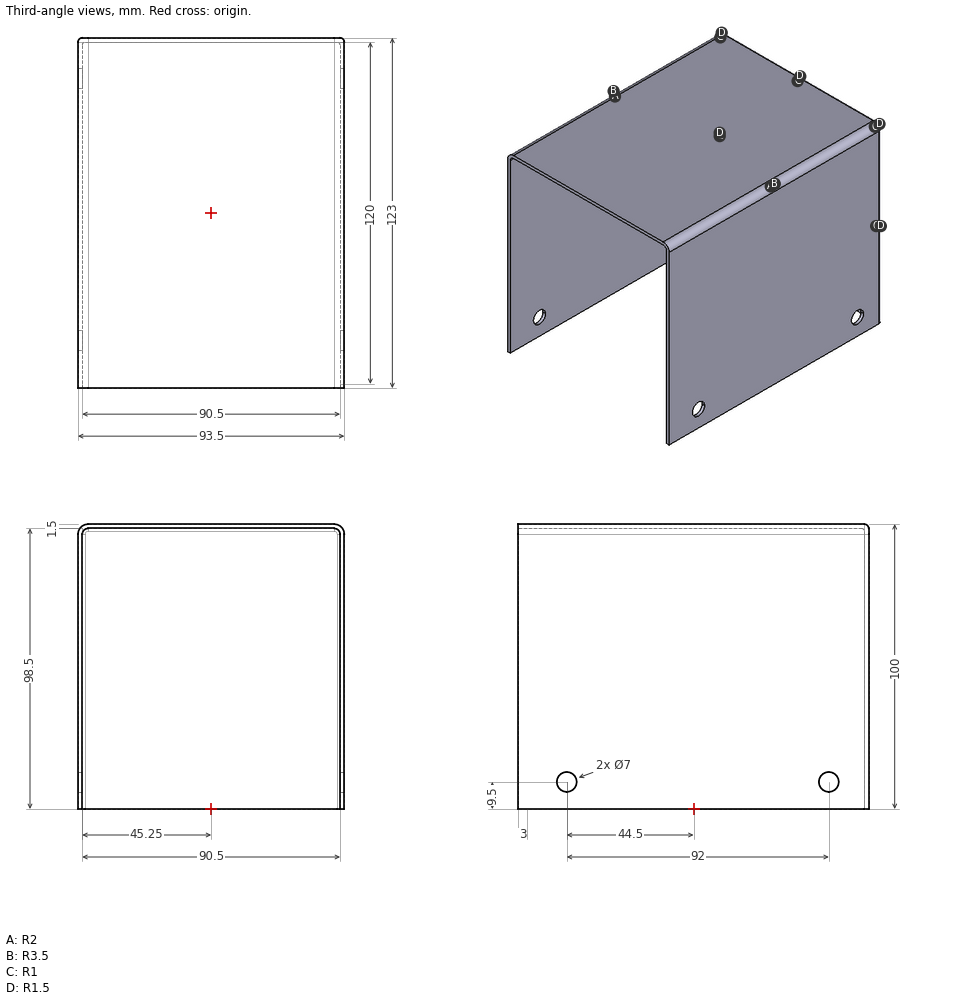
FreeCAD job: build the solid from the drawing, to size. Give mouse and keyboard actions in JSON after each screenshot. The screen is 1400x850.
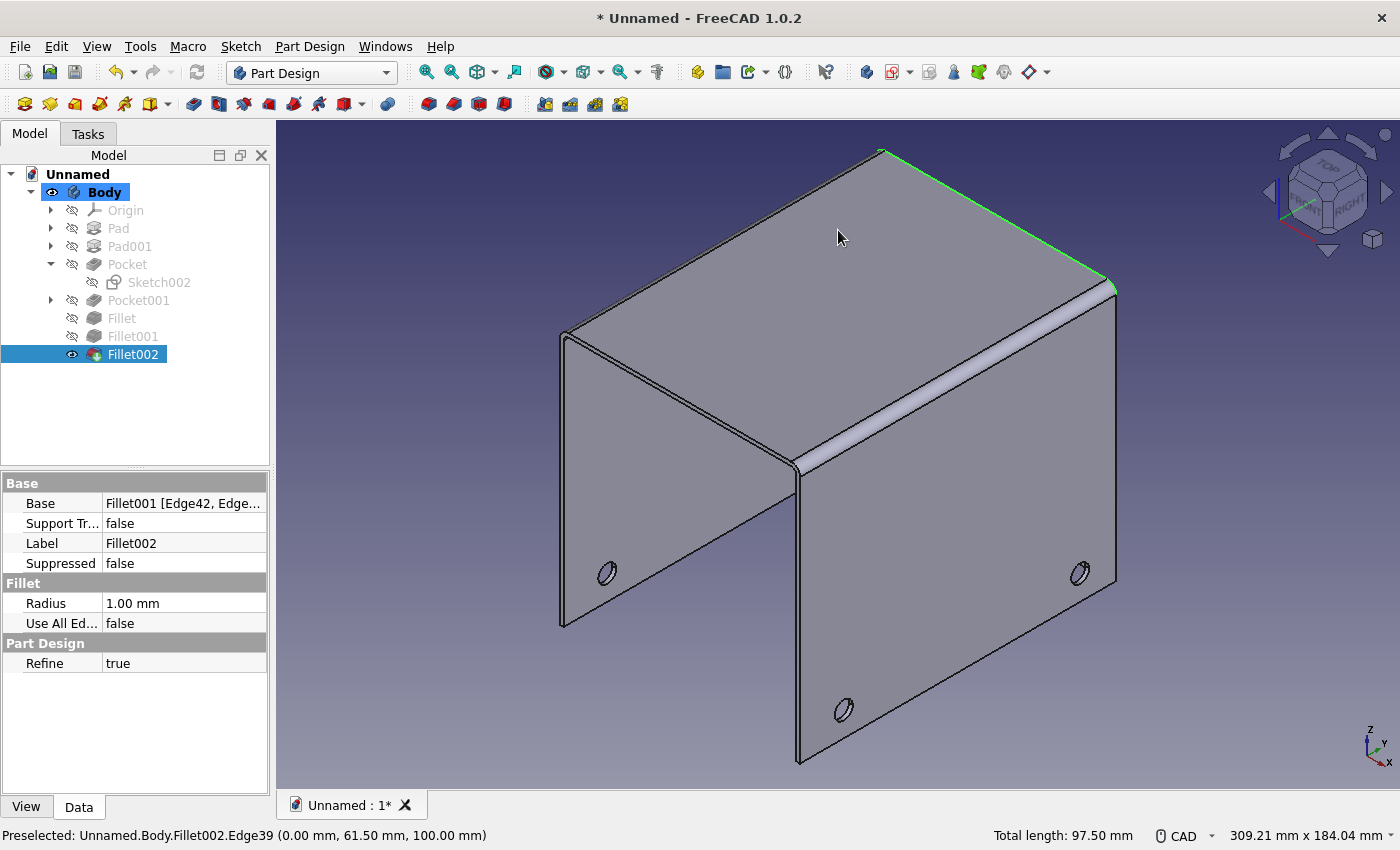
{"action": "key", "text": "1"}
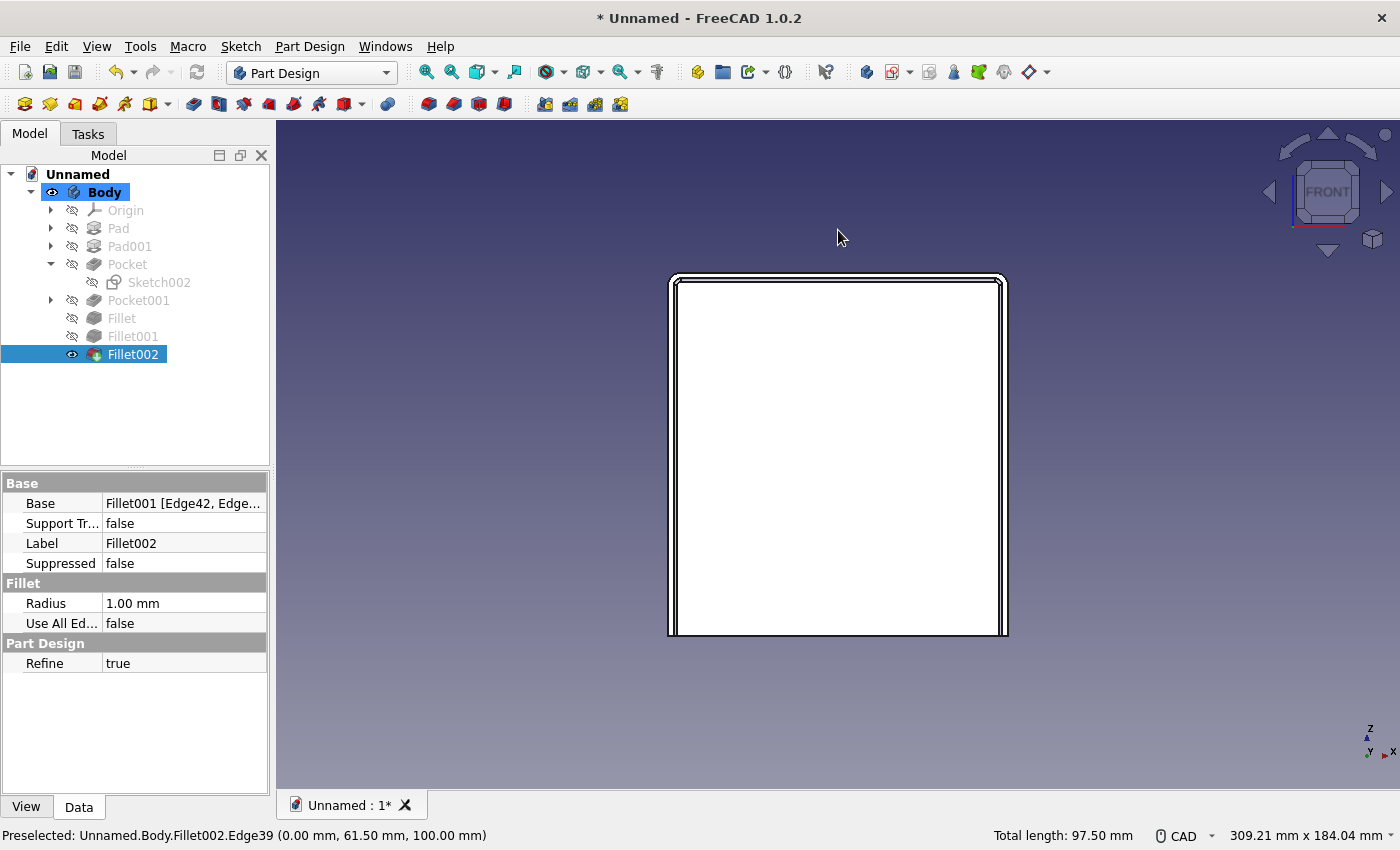
{"action": "key", "text": "3"}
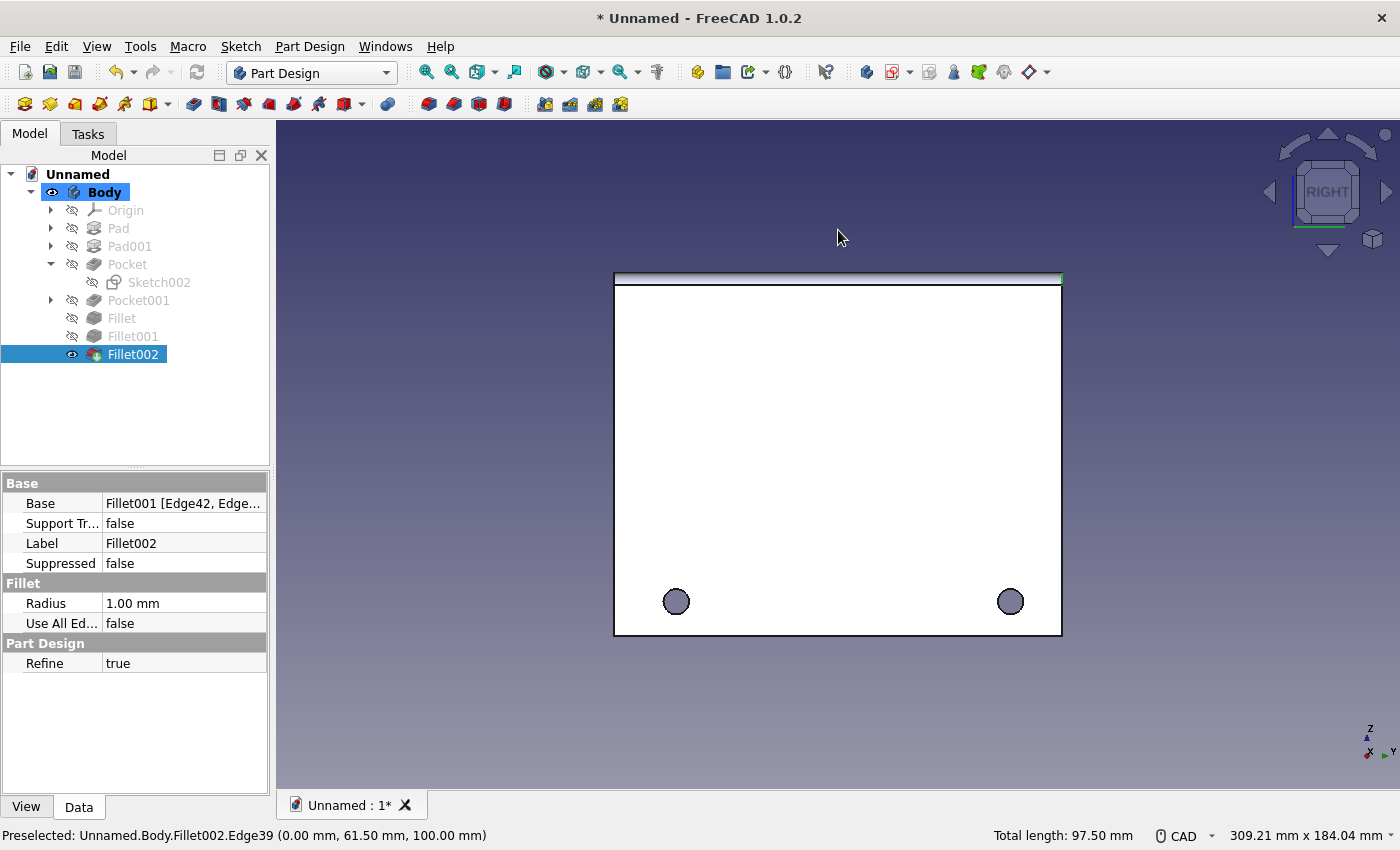
{"action": "left_click", "coordinate": [1062, 460], "text": "ctrl"}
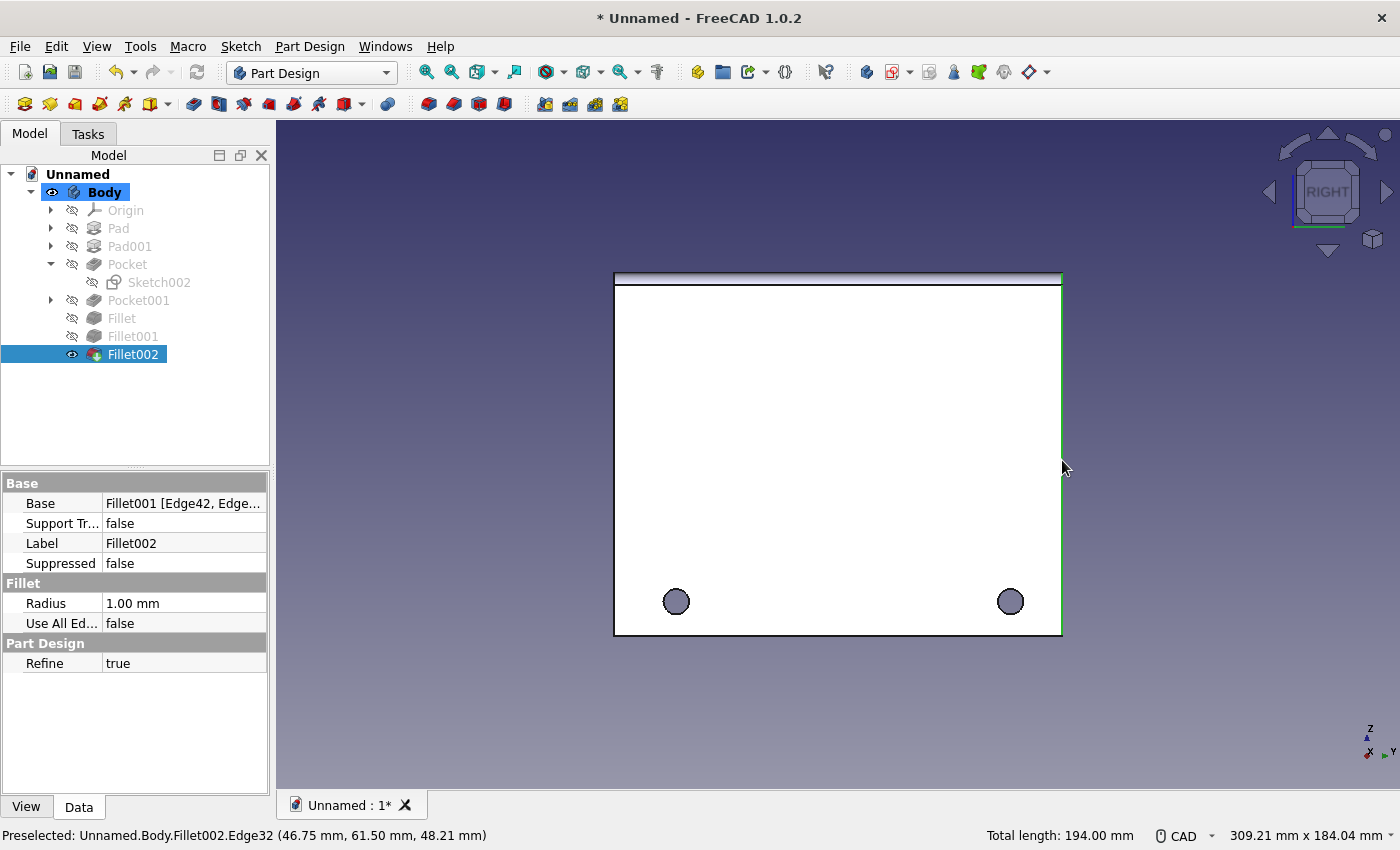
{"action": "key", "text": "5"}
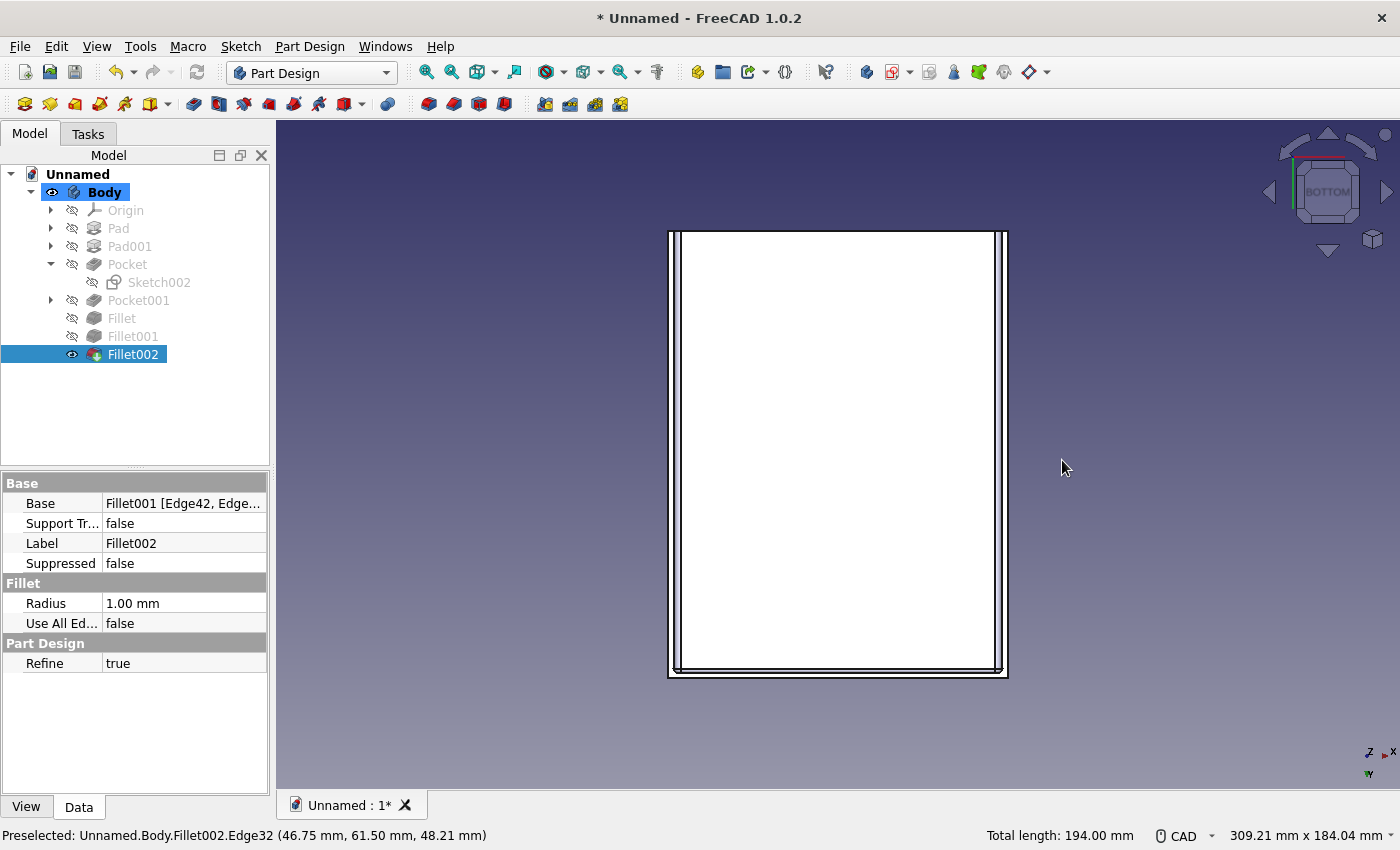
{"action": "key", "text": "4"}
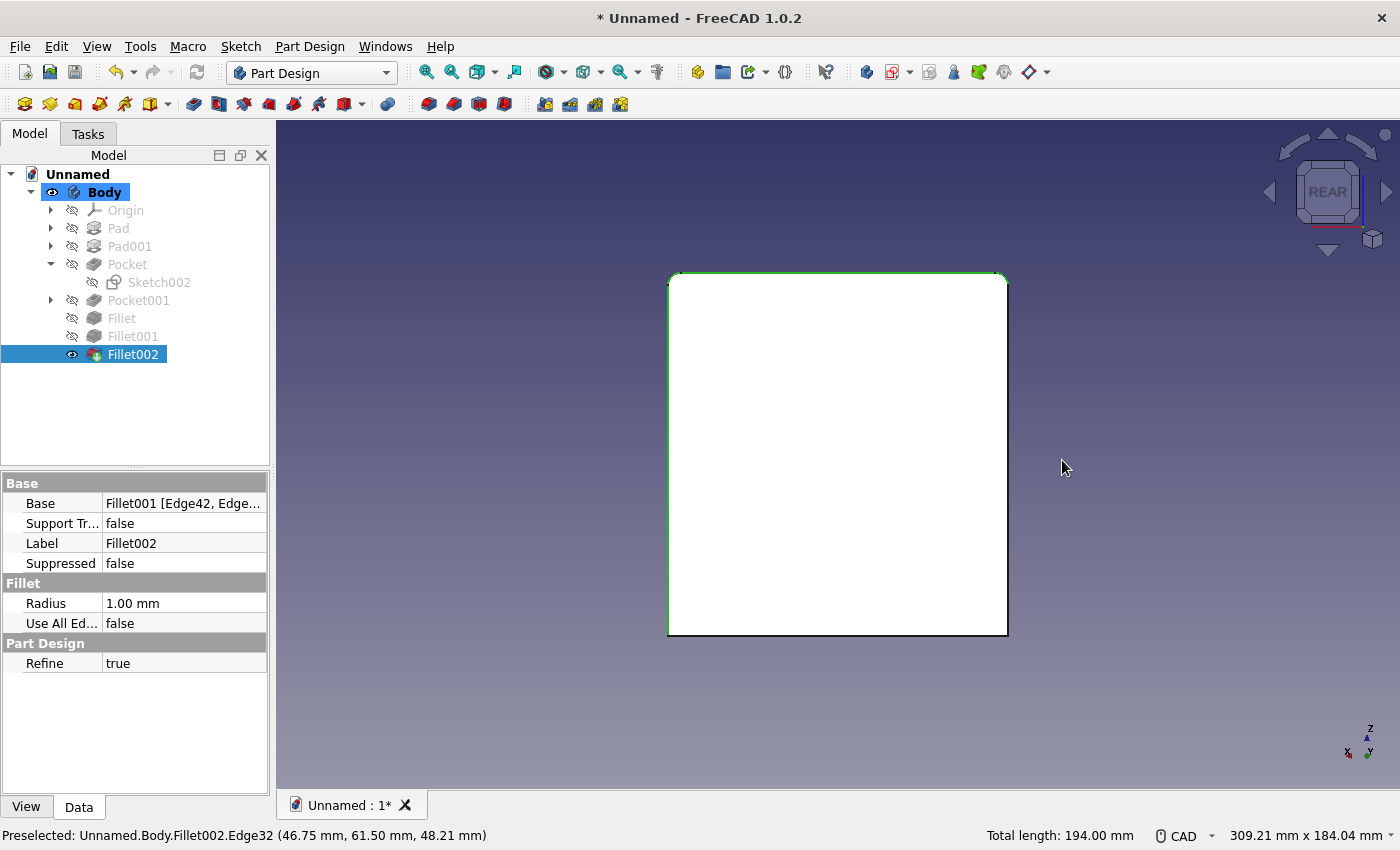
{"action": "left_click", "coordinate": [1008, 460], "text": "ctrl"}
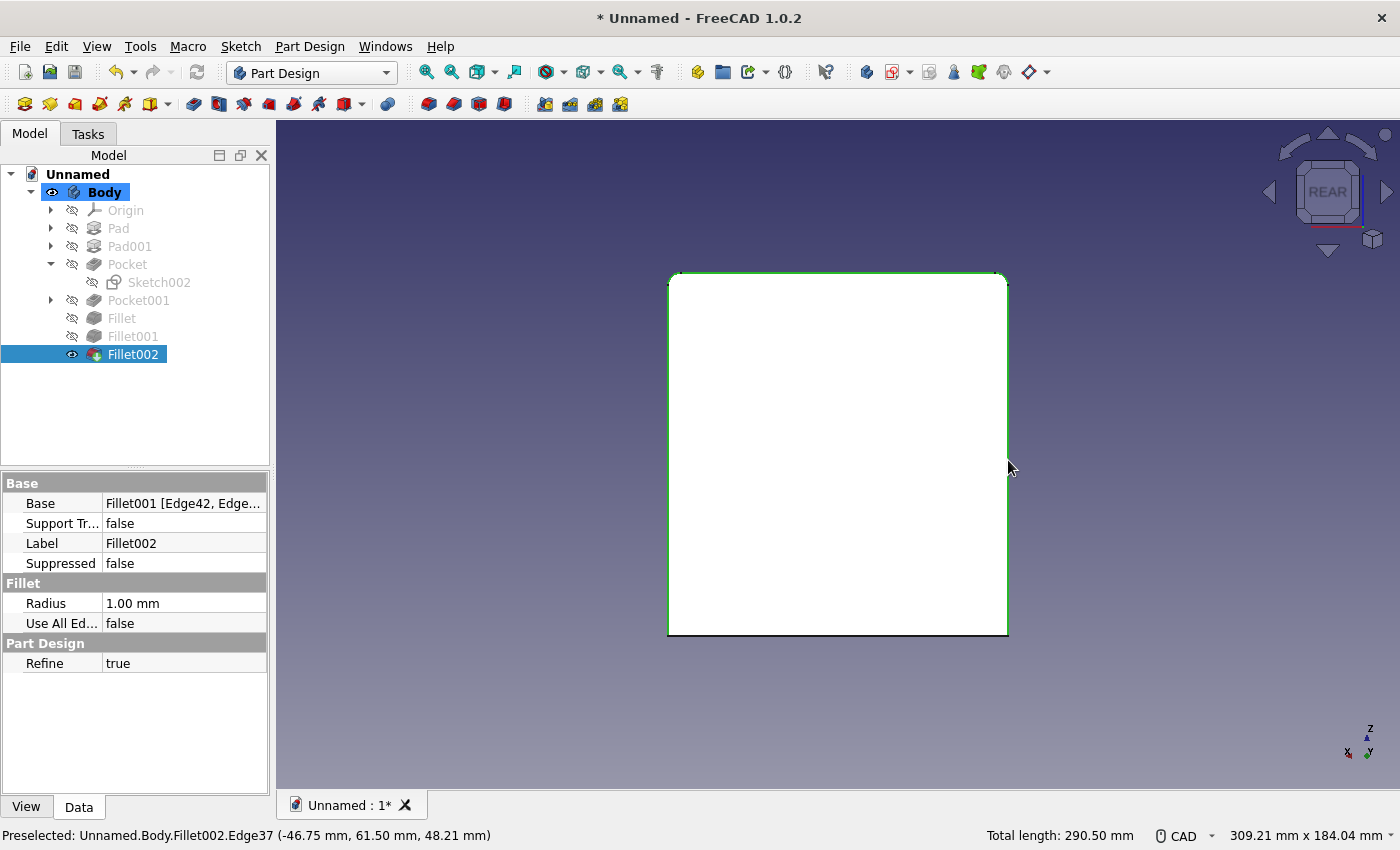
{"action": "left_click", "coordinate": [429, 104]}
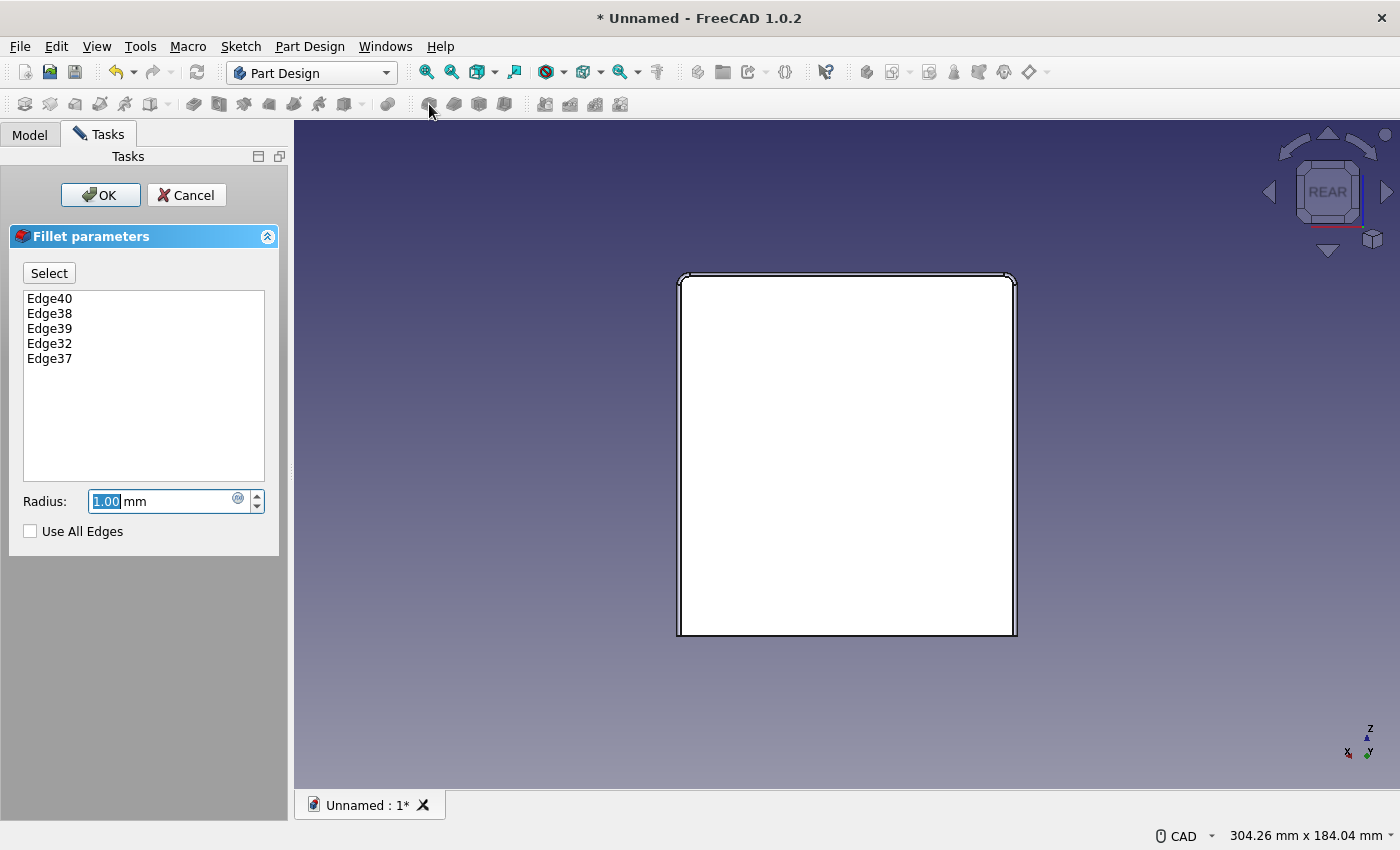
{"action": "type", "text": "1.5"}
{"action": "key", "text": "Tab"}